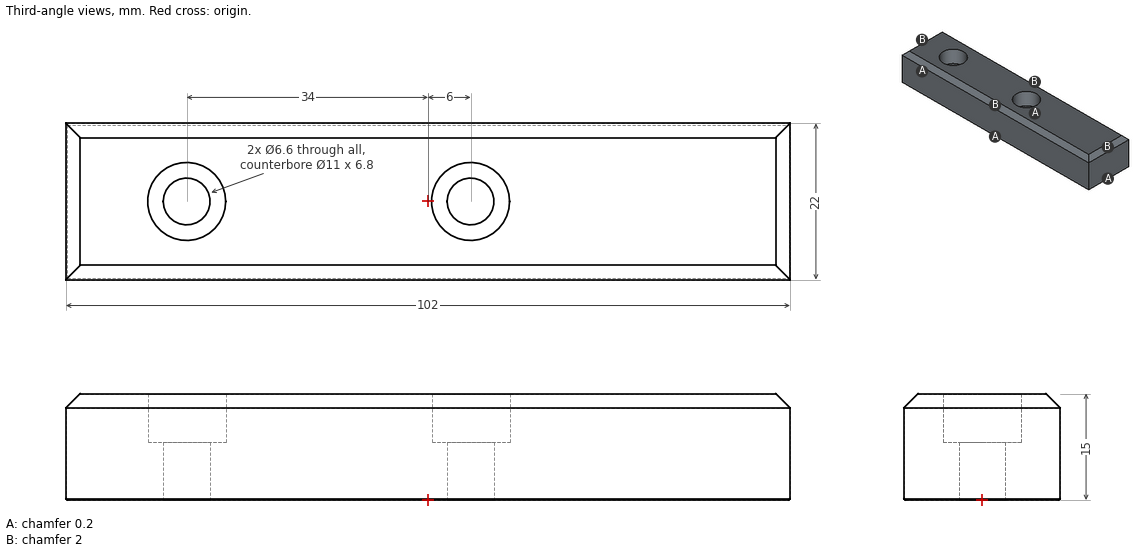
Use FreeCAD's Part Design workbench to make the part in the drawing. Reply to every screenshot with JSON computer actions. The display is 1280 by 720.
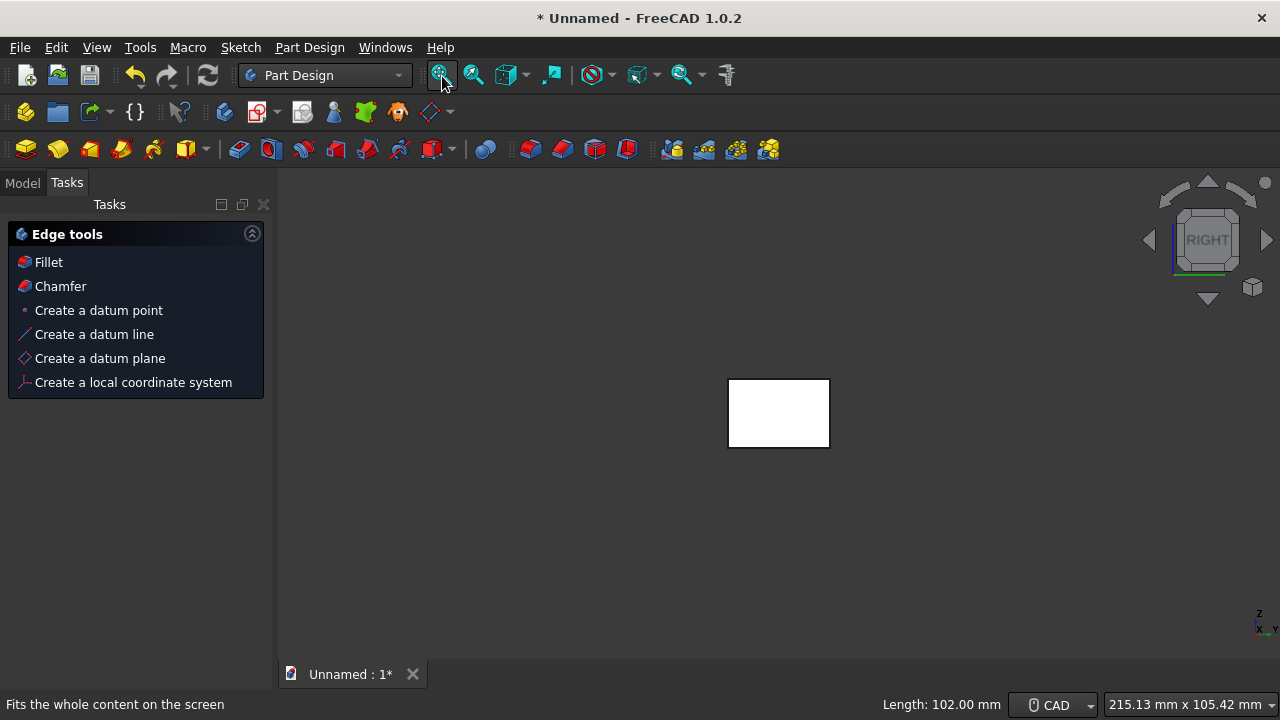
{"action": "left_click", "coordinate": [779, 447], "text": "ctrl"}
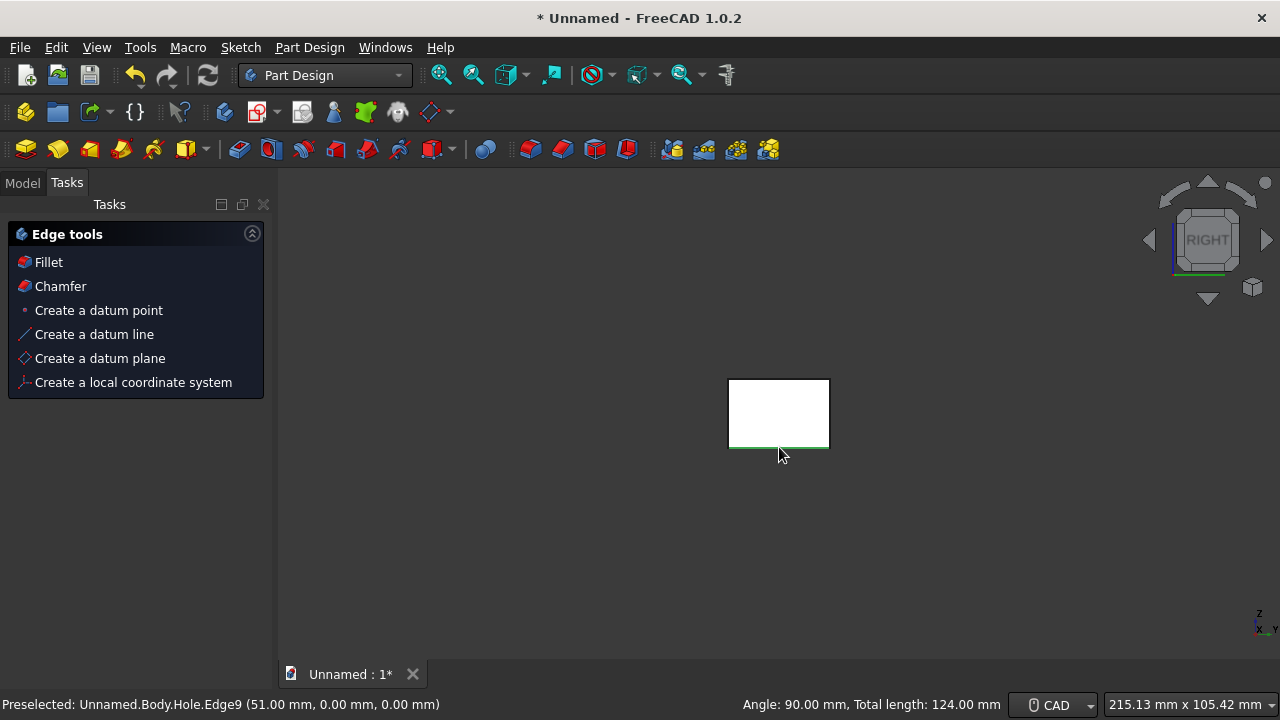
{"action": "key", "text": "5"}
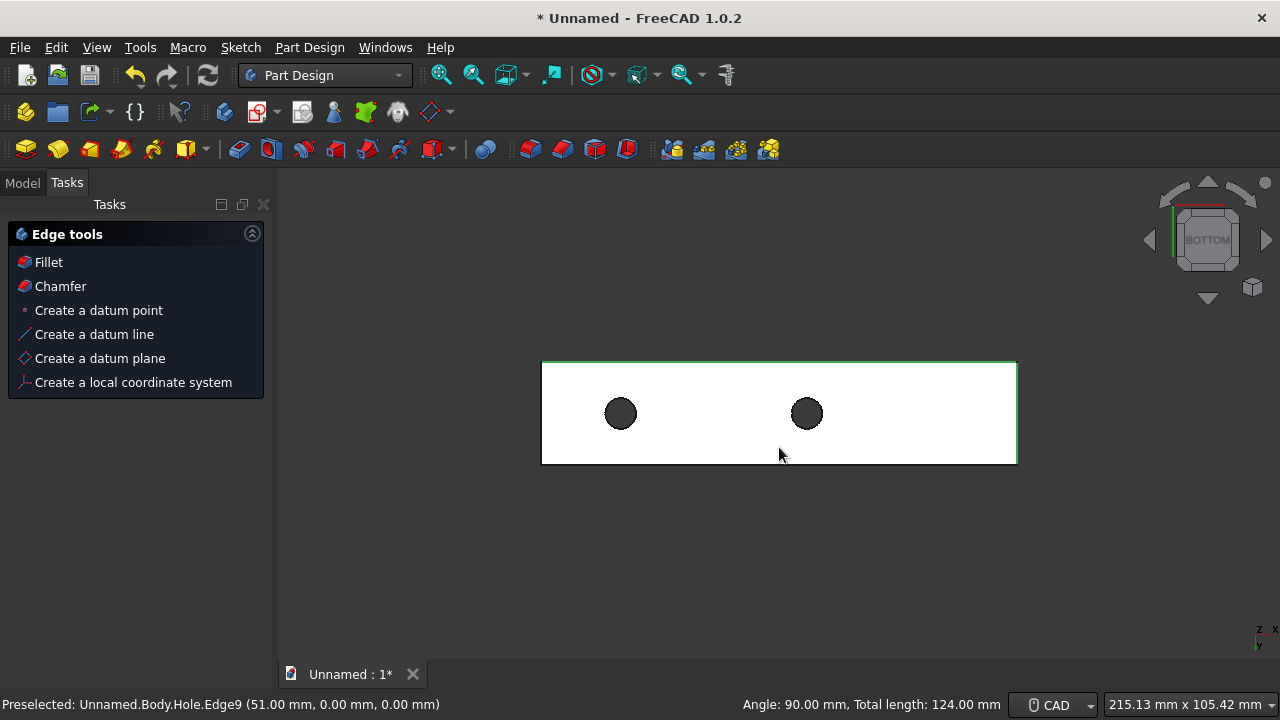
{"action": "left_click", "coordinate": [779, 464], "text": "ctrl"}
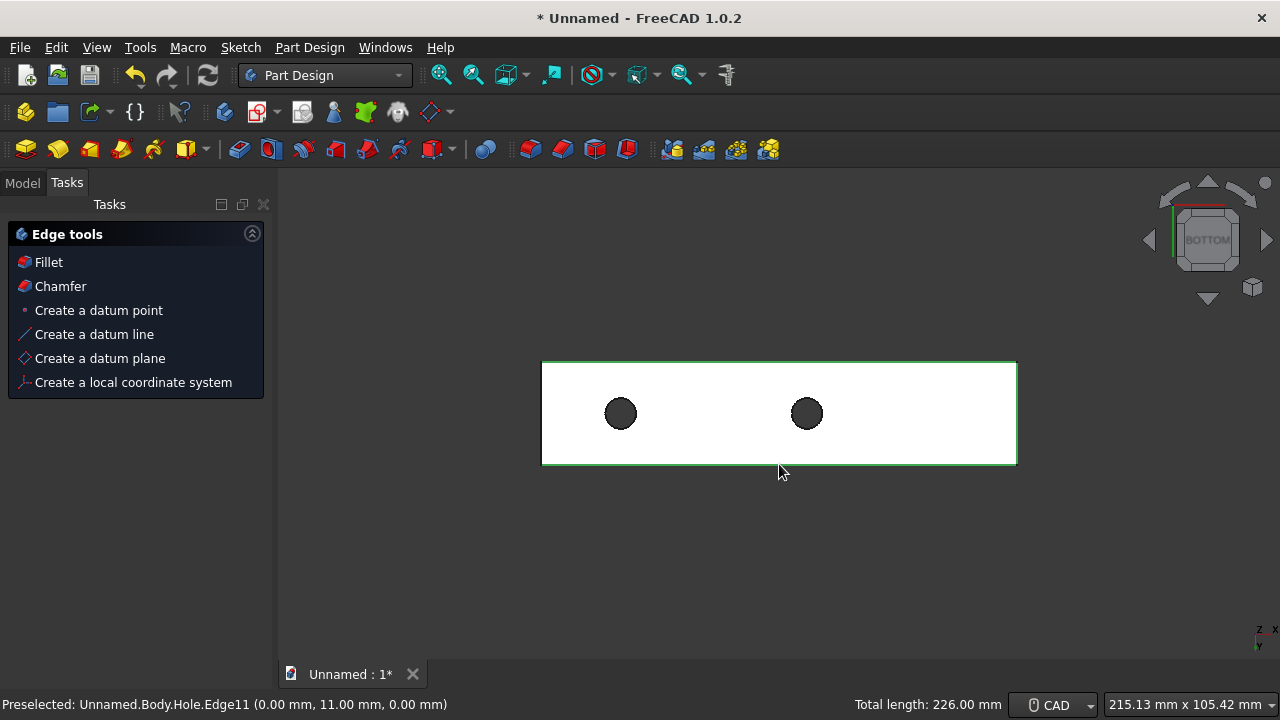
{"action": "left_click", "coordinate": [541, 412], "text": "ctrl"}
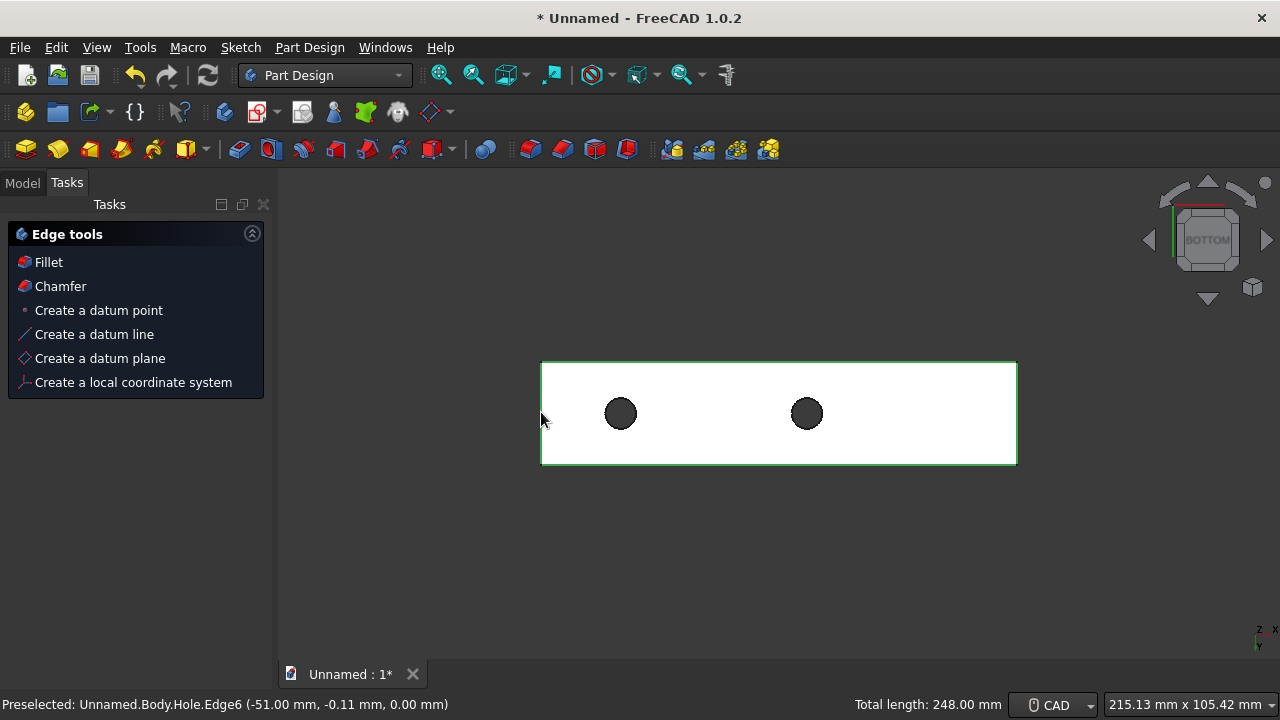
{"action": "left_click", "coordinate": [564, 150]}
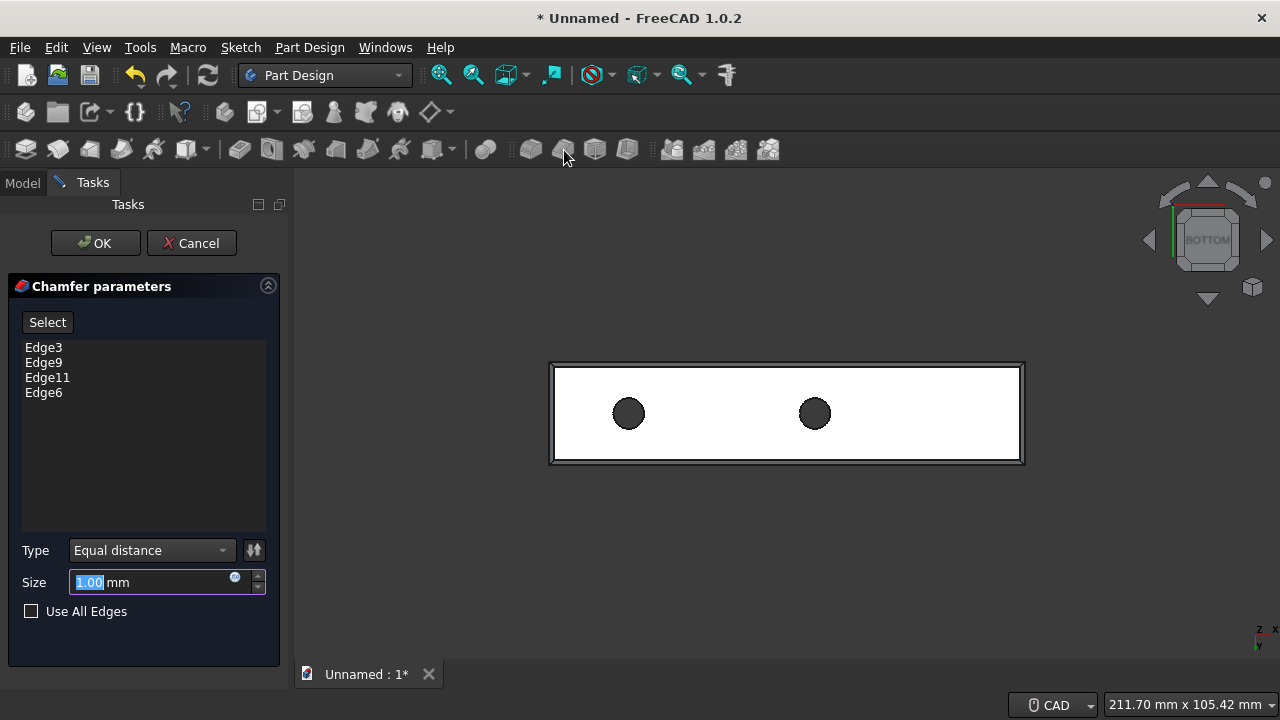
{"action": "type", "text": "0.2"}
{"action": "key", "text": "Tab"}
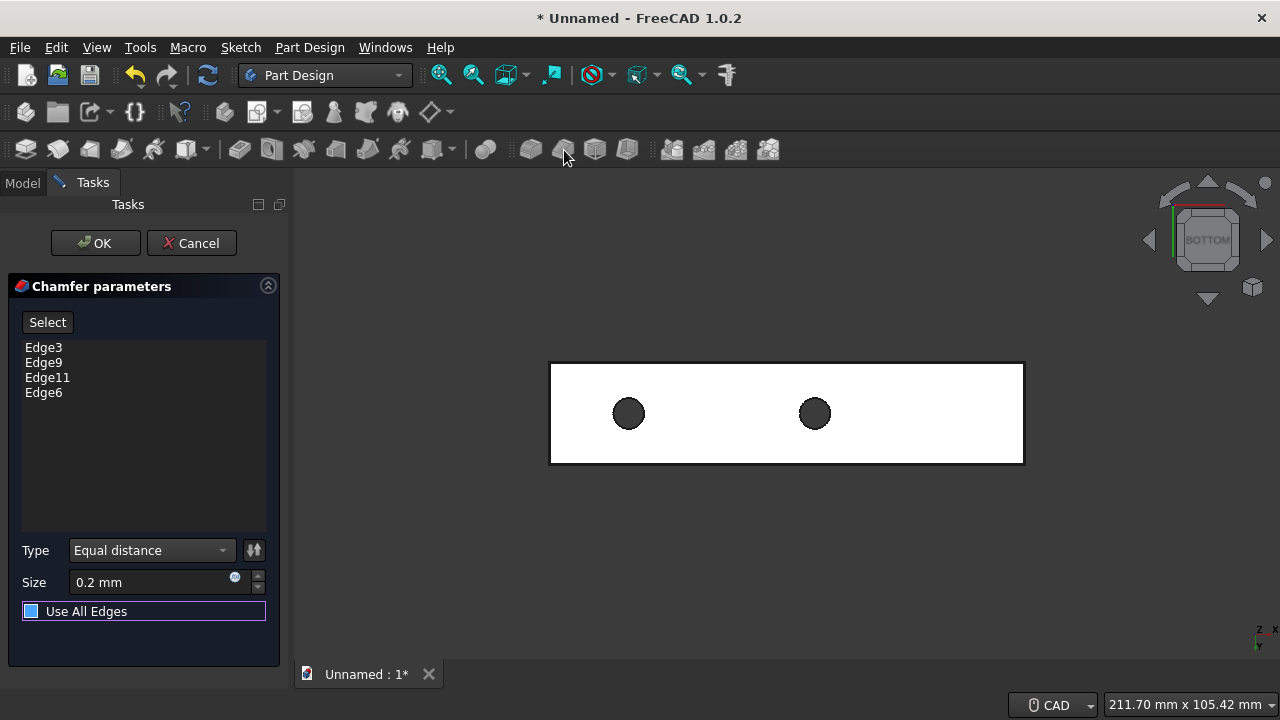
{"action": "left_click", "coordinate": [96, 243]}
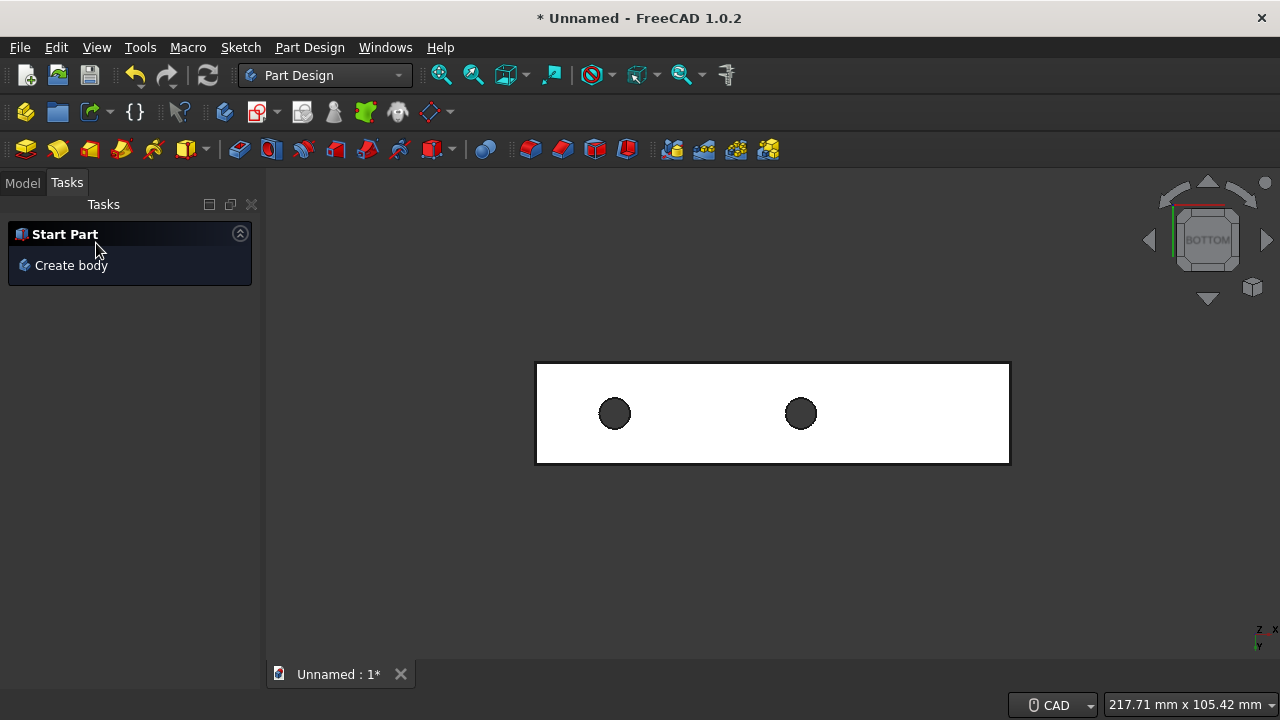
{"action": "key", "text": "0"}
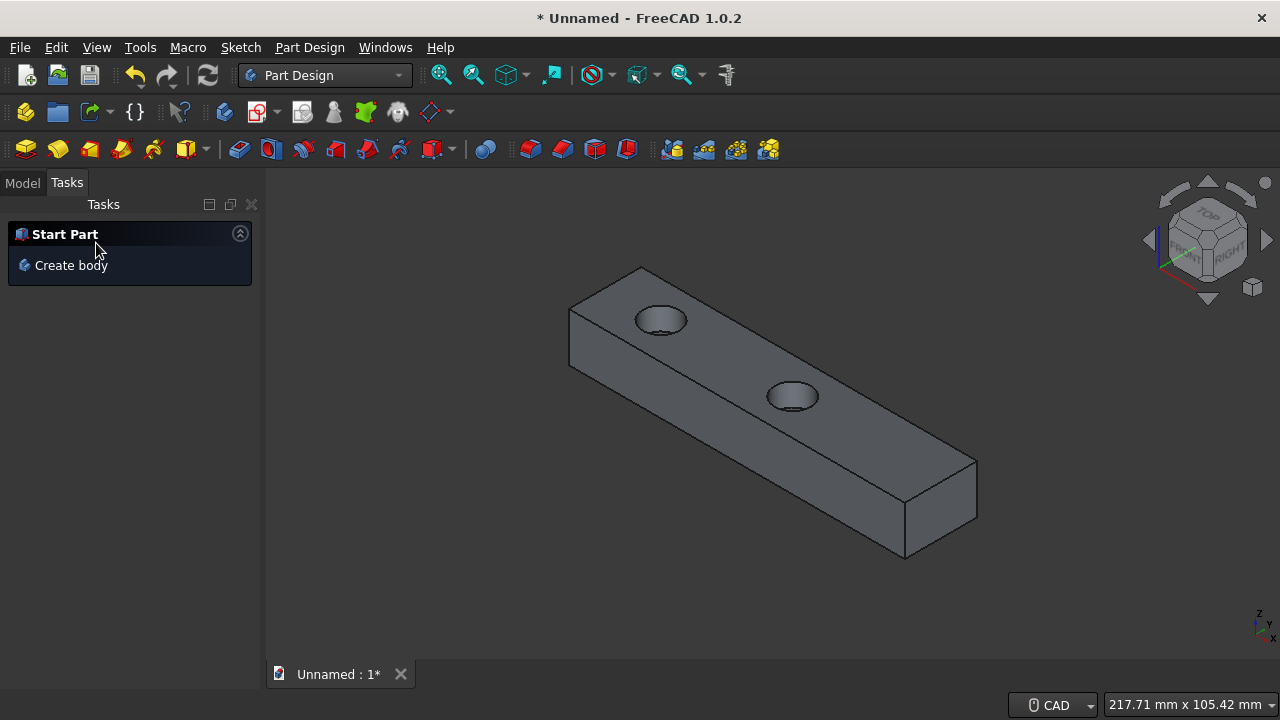
{"action": "left_click", "coordinate": [941, 481]}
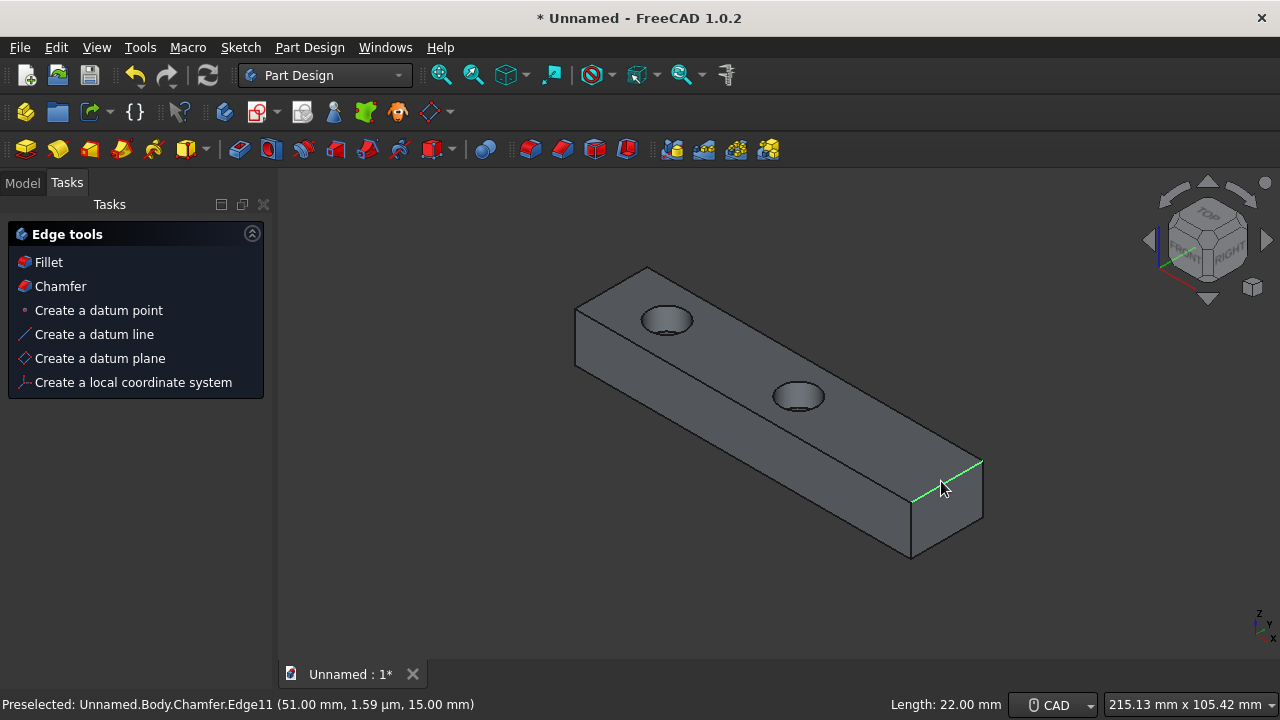
{"action": "left_click", "coordinate": [743, 405], "text": "ctrl"}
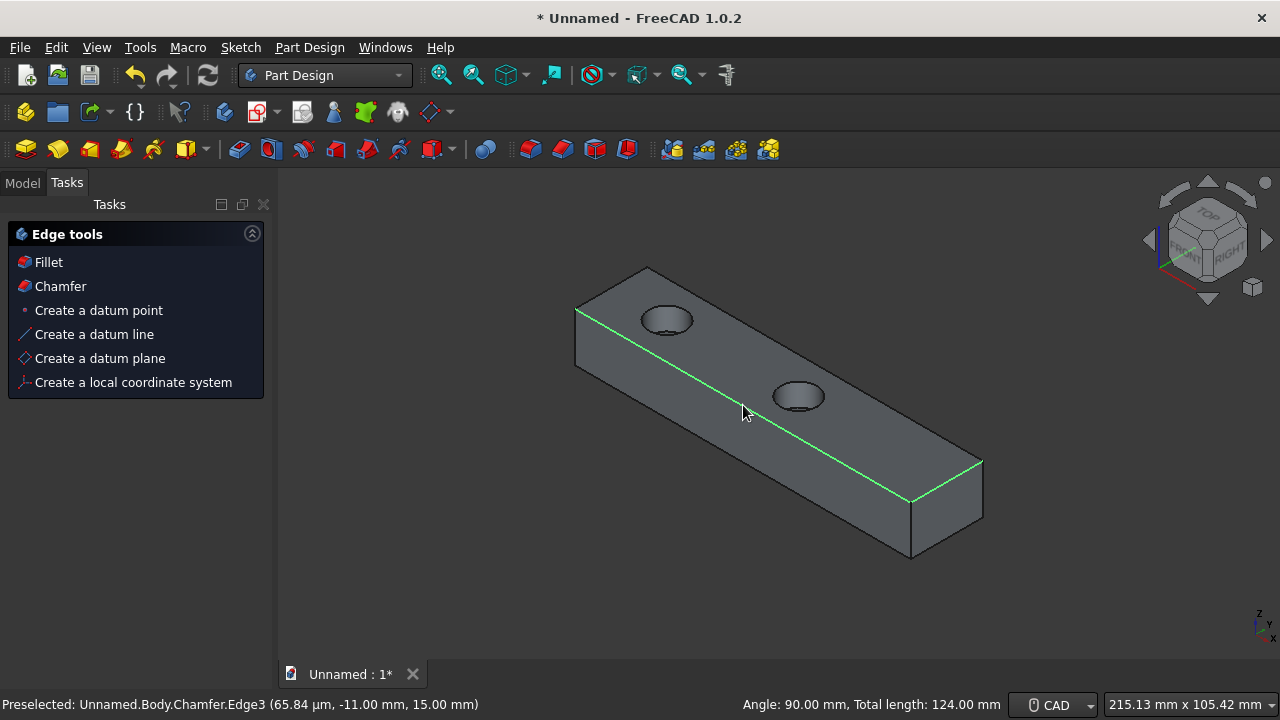
{"action": "key", "text": "2"}